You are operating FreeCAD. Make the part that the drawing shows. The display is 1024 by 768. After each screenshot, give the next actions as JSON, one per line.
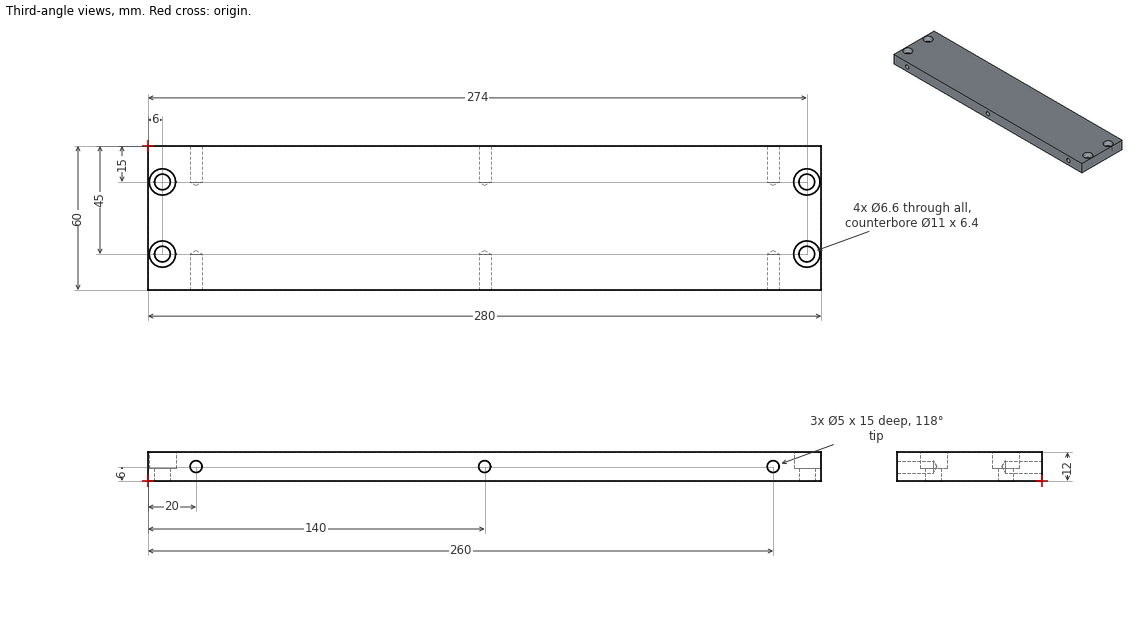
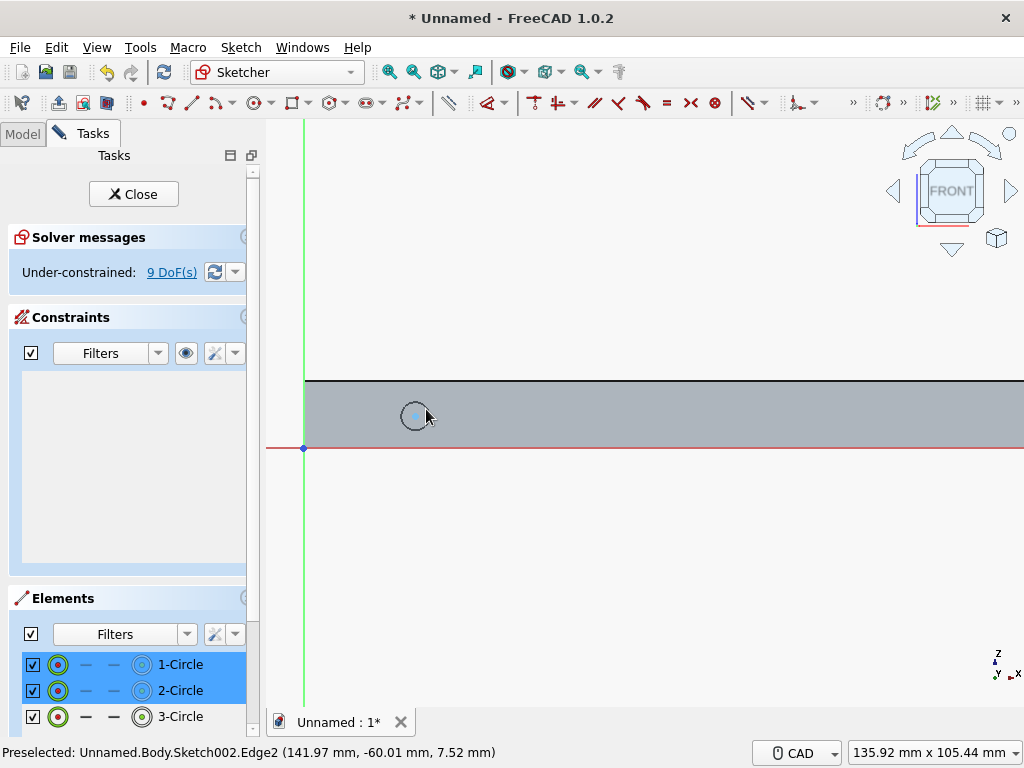
{"action": "left_click", "coordinate": [425, 406]}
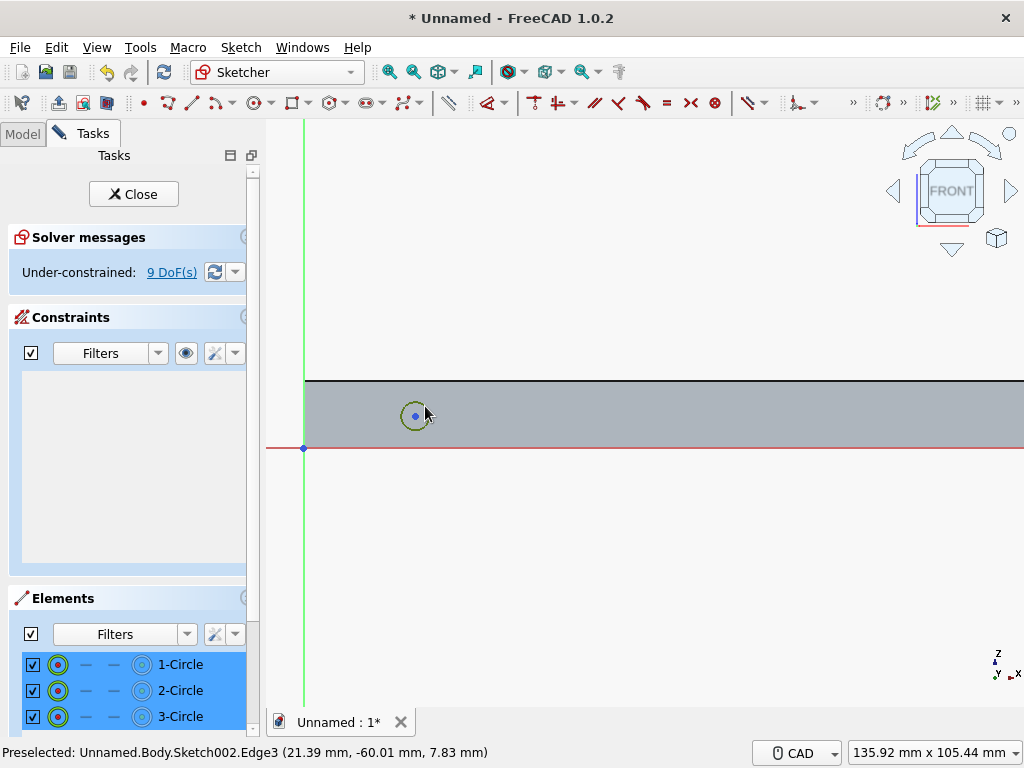
{"action": "left_click", "coordinate": [668, 104]}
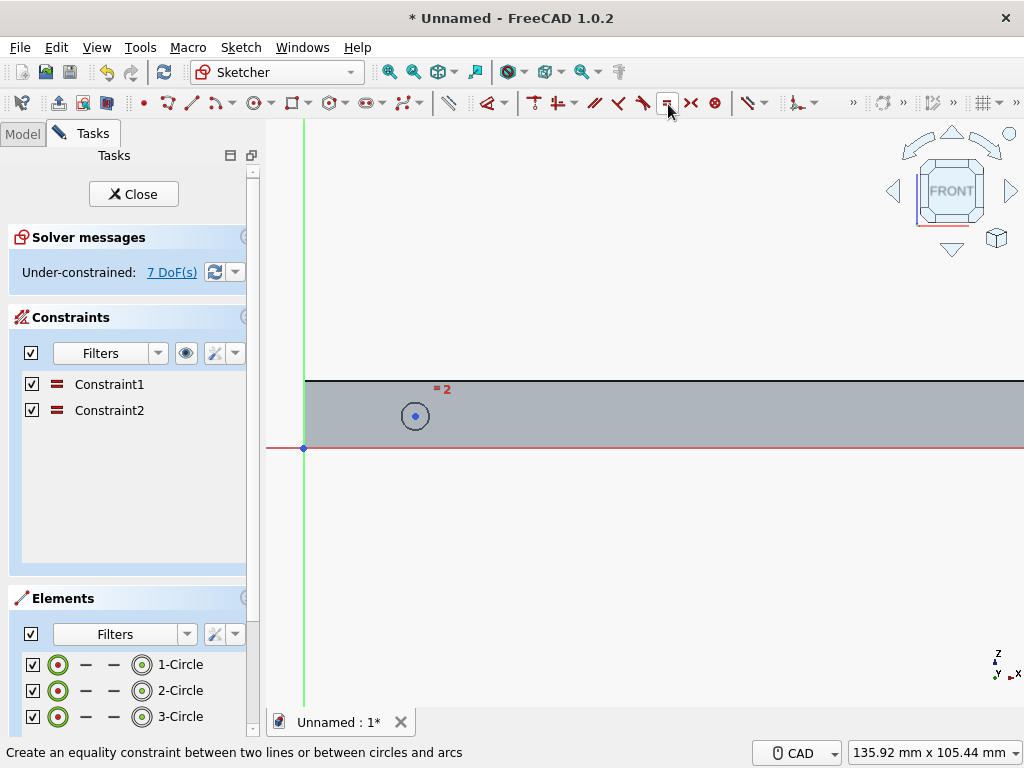
{"action": "left_click", "coordinate": [488, 104]}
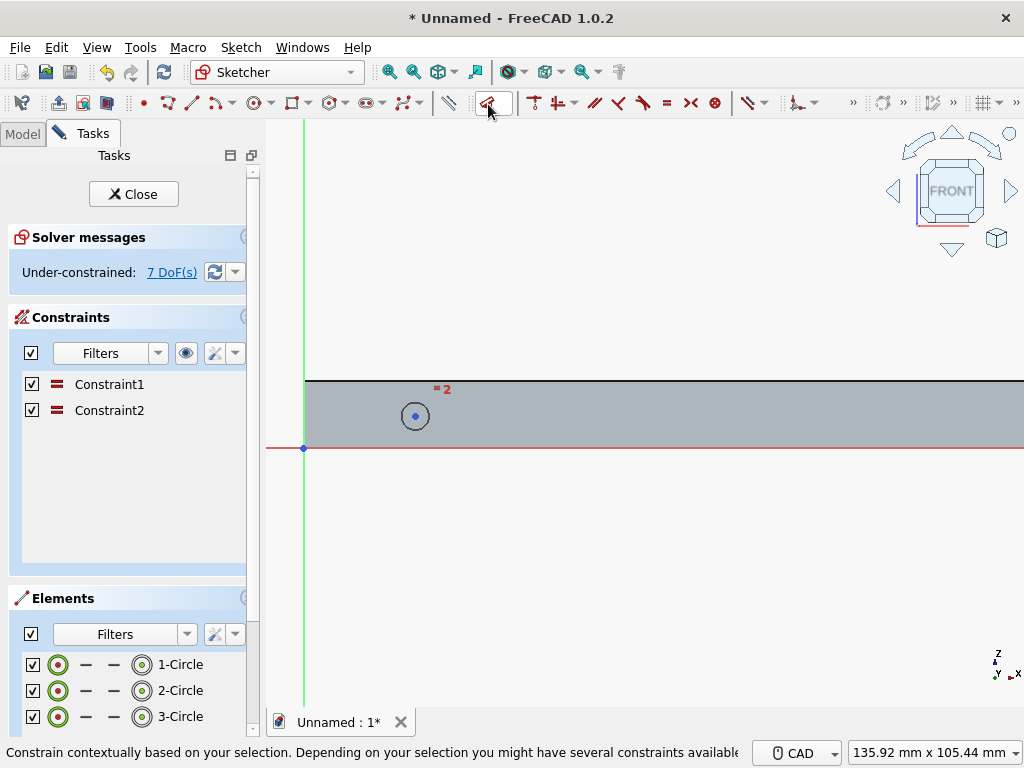
{"action": "scroll", "coordinate": [426, 409], "scroll_direction": "down", "scroll_amount": 7}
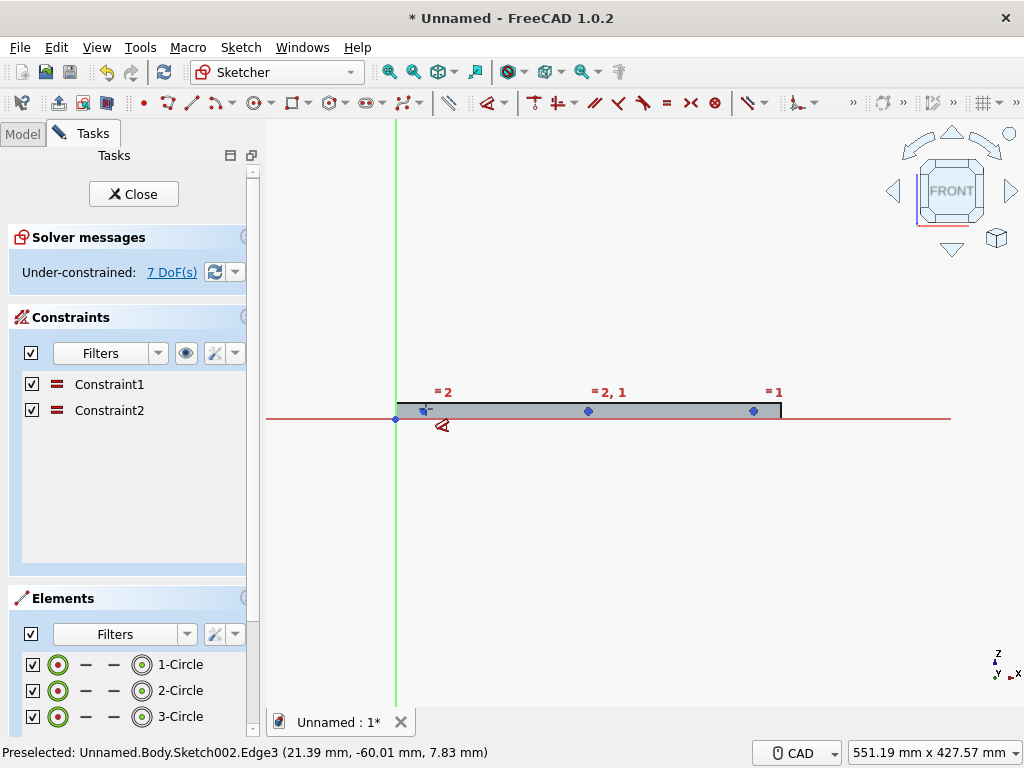
{"action": "scroll", "coordinate": [756, 409], "scroll_direction": "up", "scroll_amount": 9}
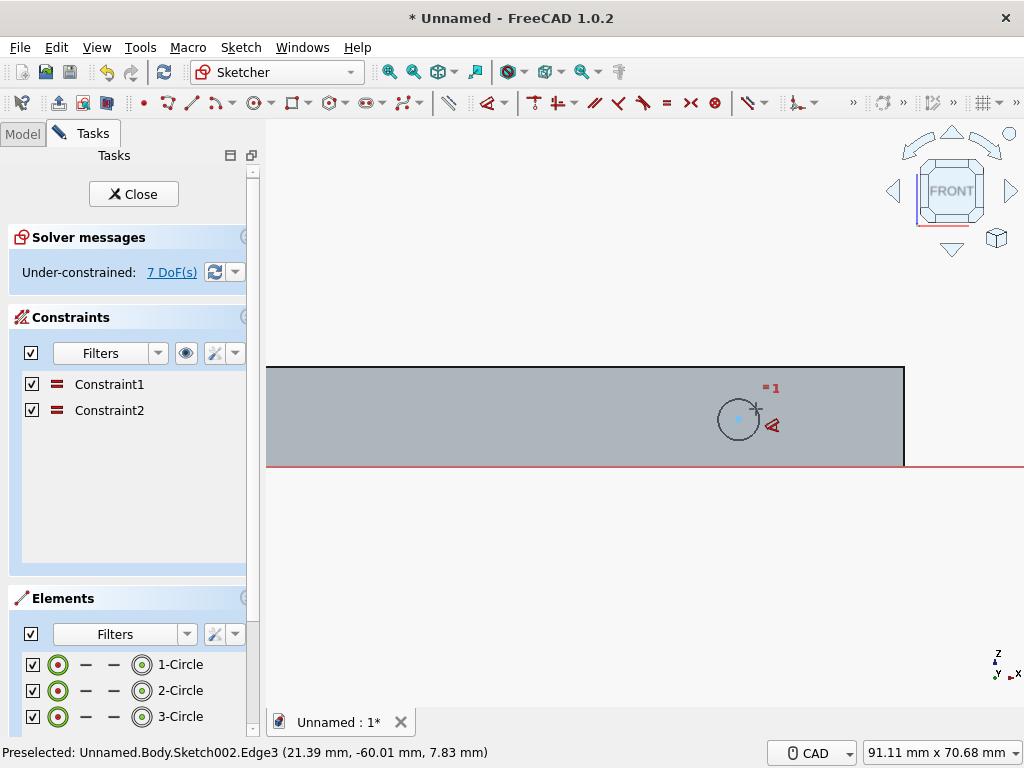
{"action": "left_click", "coordinate": [753, 405]}
{"action": "left_click", "coordinate": [775, 382]}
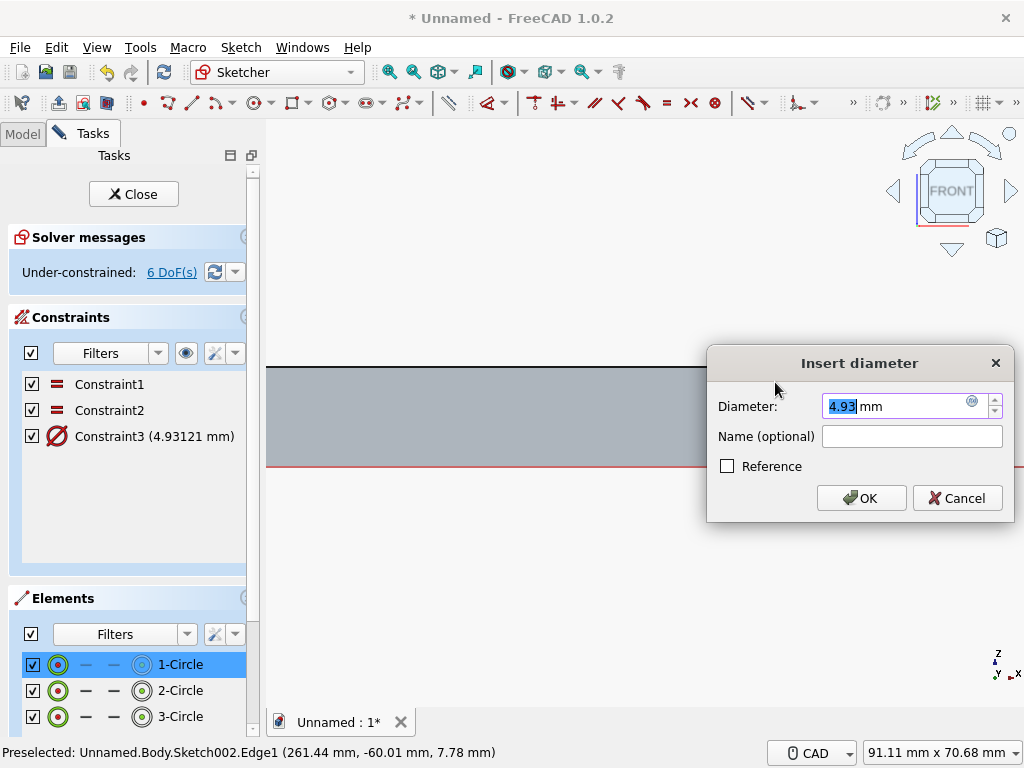
{"action": "type", "text": "5"}
{"action": "key", "text": "Return"}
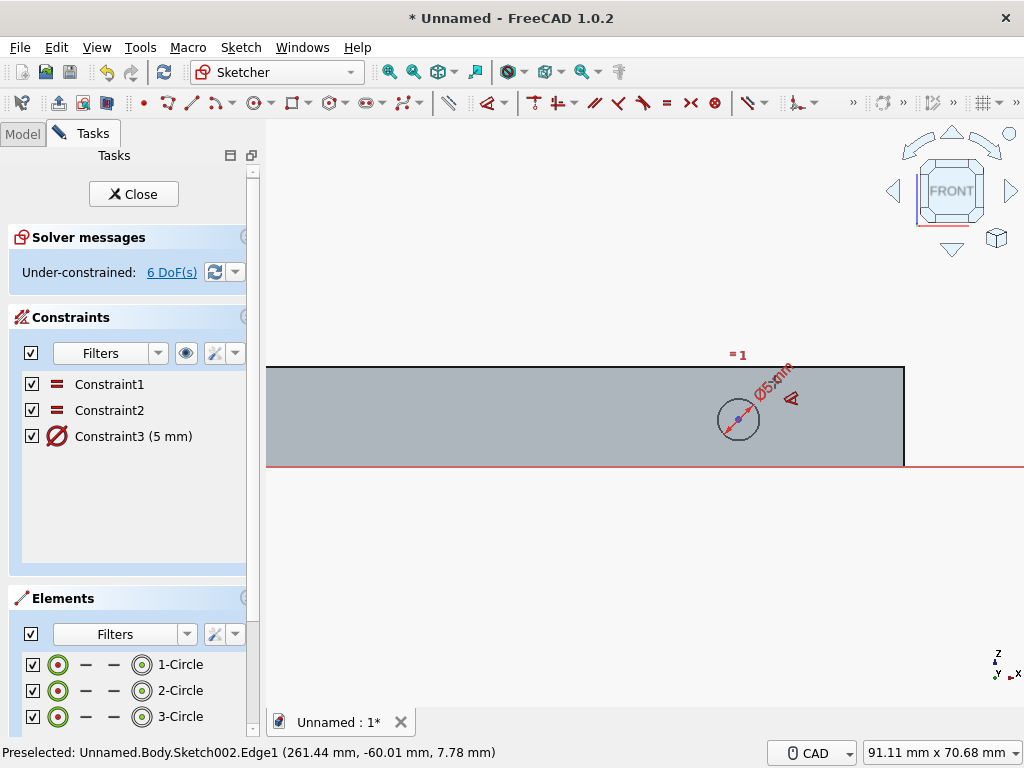
{"action": "left_click", "coordinate": [739, 420]}
{"action": "left_click", "coordinate": [773, 443]}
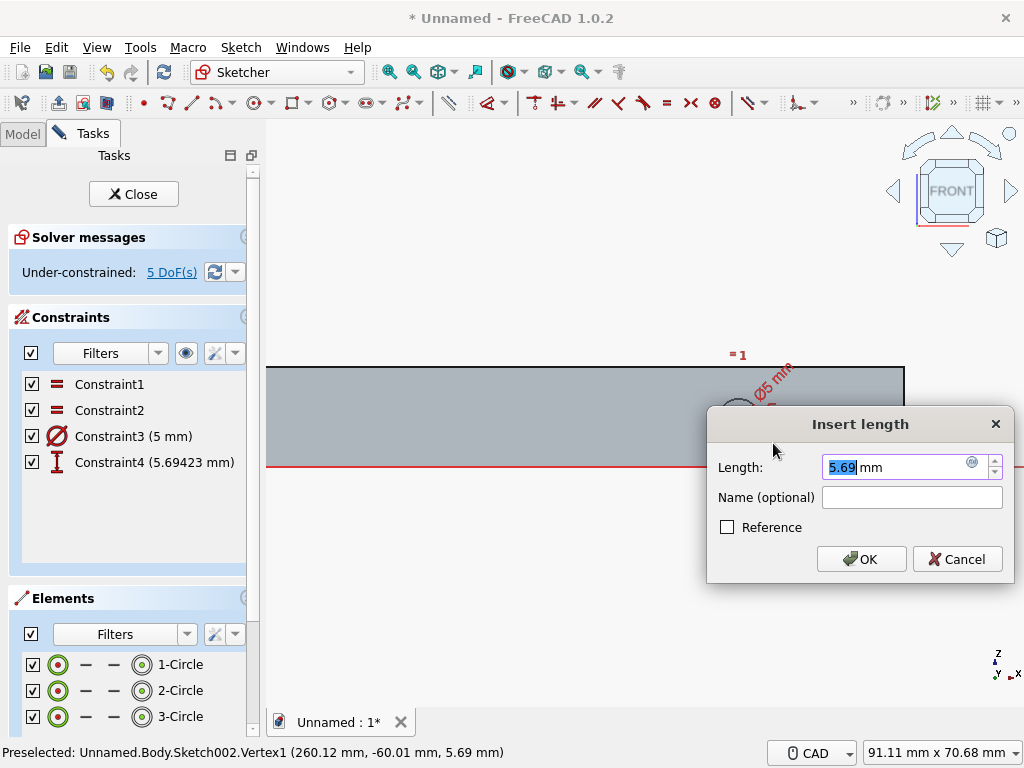
{"action": "type", "text": "6"}
{"action": "key", "text": "Return"}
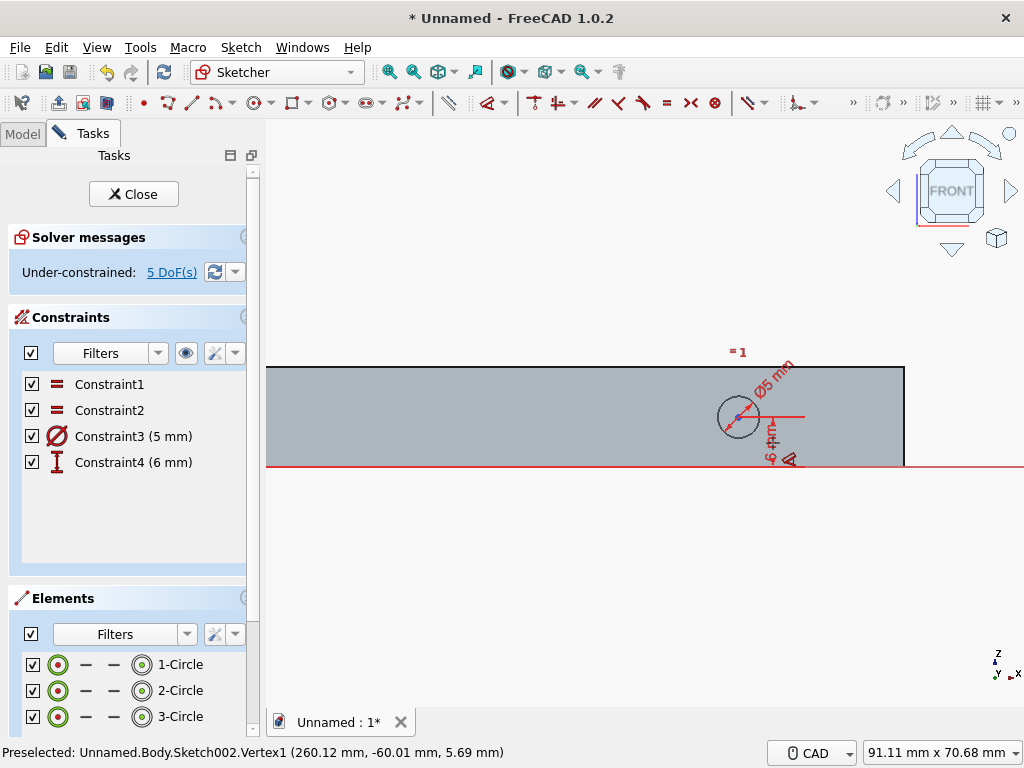
{"action": "scroll", "coordinate": [757, 409], "scroll_direction": "down", "scroll_amount": 9}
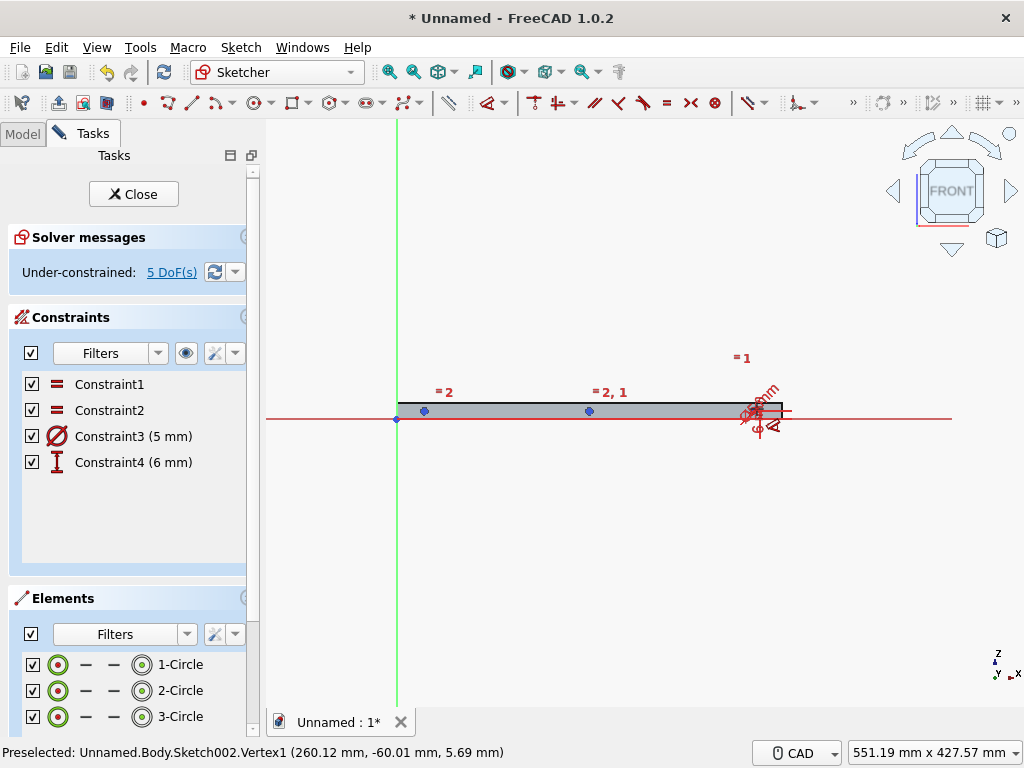
{"action": "scroll", "coordinate": [589, 411], "scroll_direction": "up", "scroll_amount": 8}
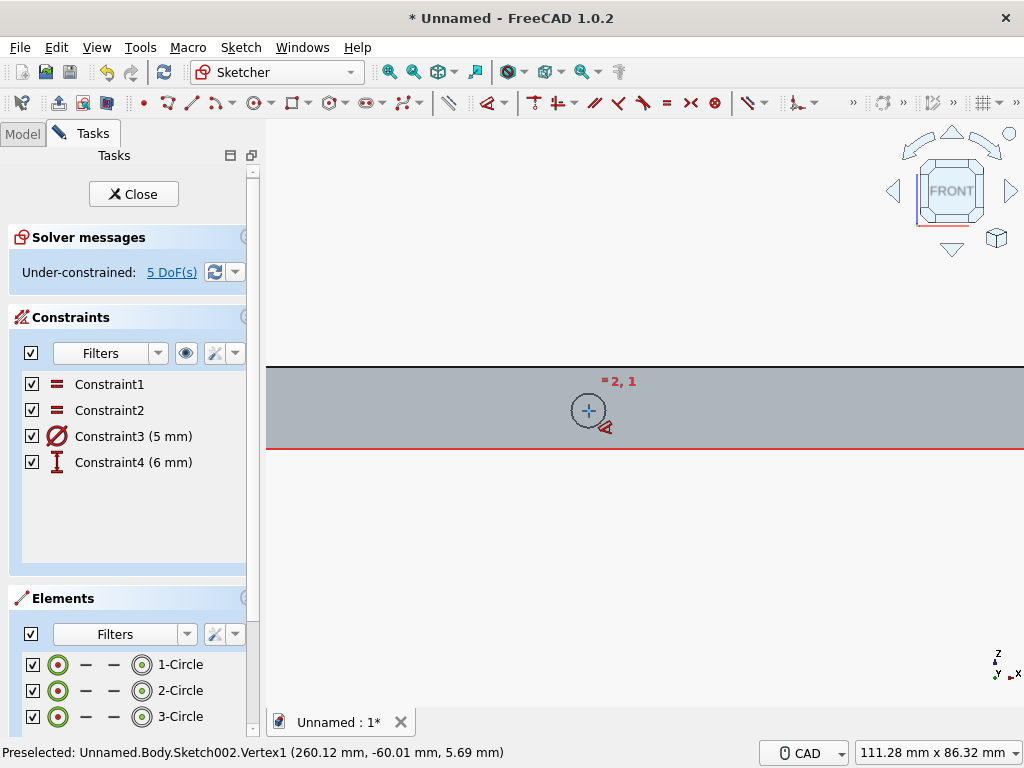
{"action": "left_click", "coordinate": [588, 411]}
{"action": "left_click", "coordinate": [622, 430]}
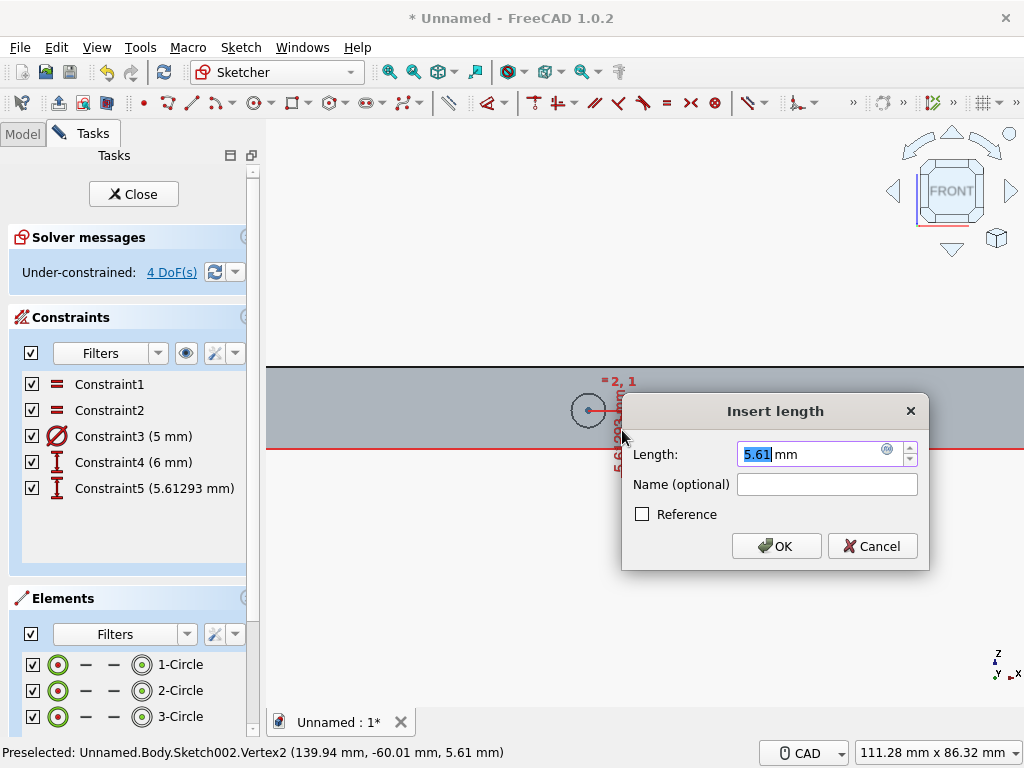
{"action": "type", "text": "6"}
{"action": "key", "text": "Return"}